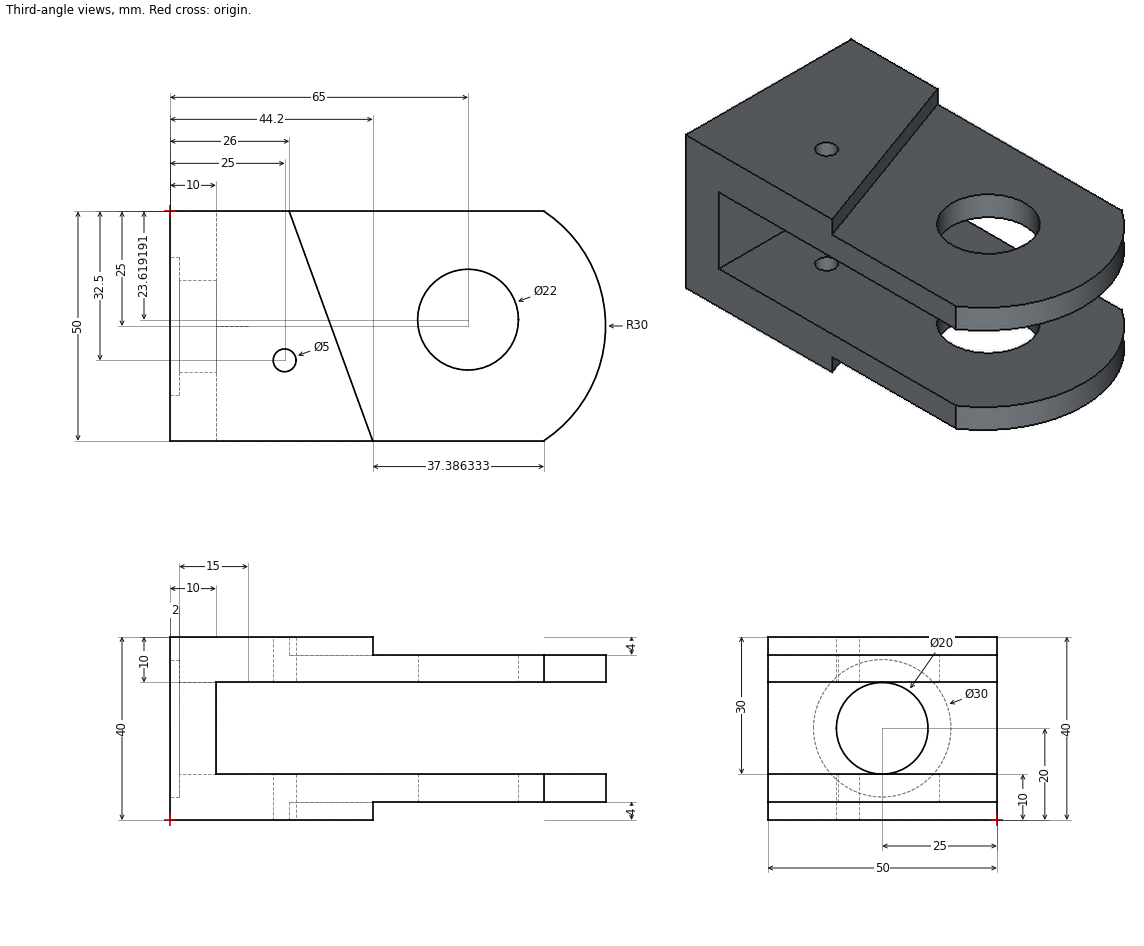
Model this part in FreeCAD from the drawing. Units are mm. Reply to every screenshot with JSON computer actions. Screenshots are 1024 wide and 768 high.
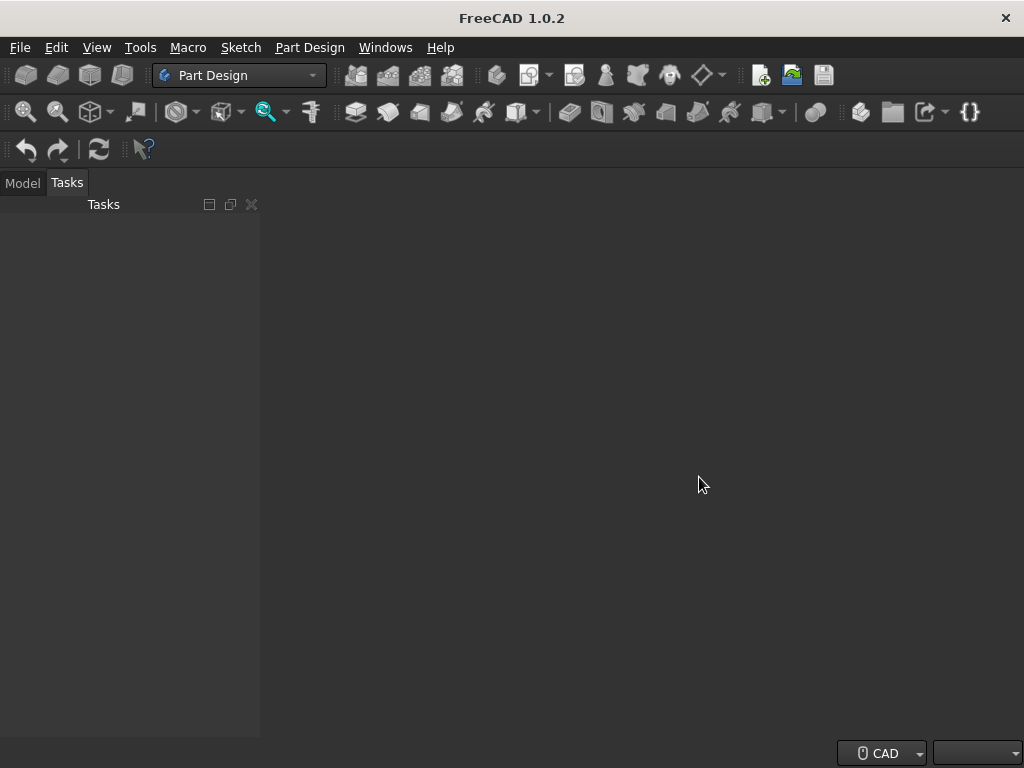
{"action": "left_click", "coordinate": [760, 76]}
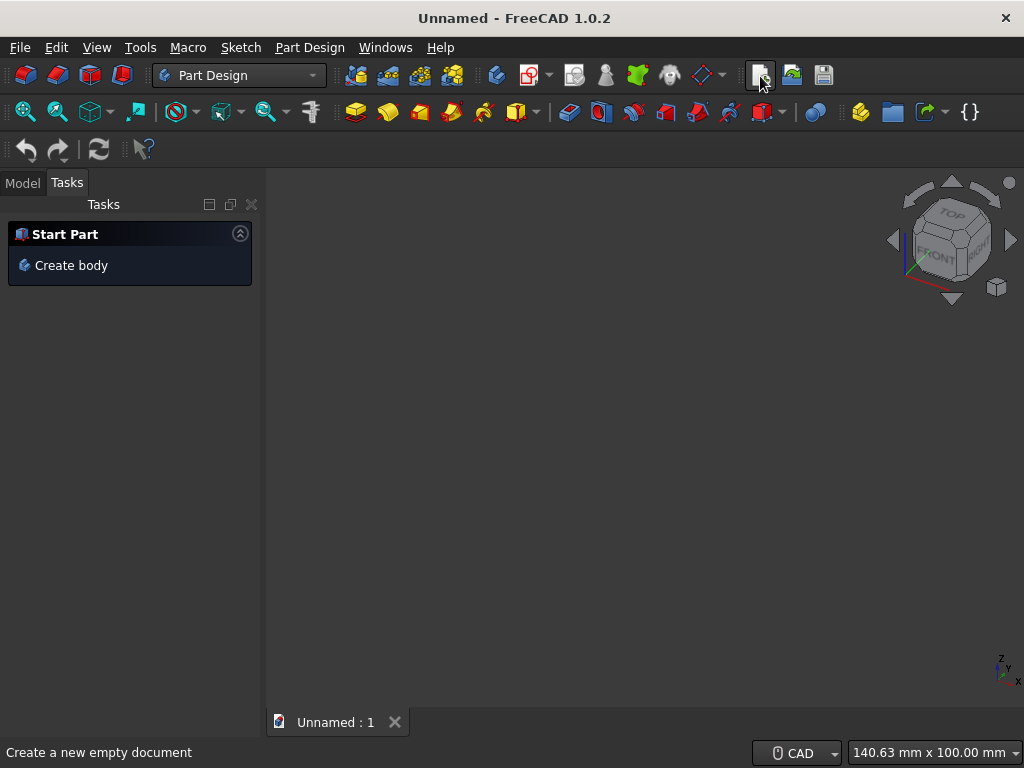
{"action": "left_click", "coordinate": [530, 76]}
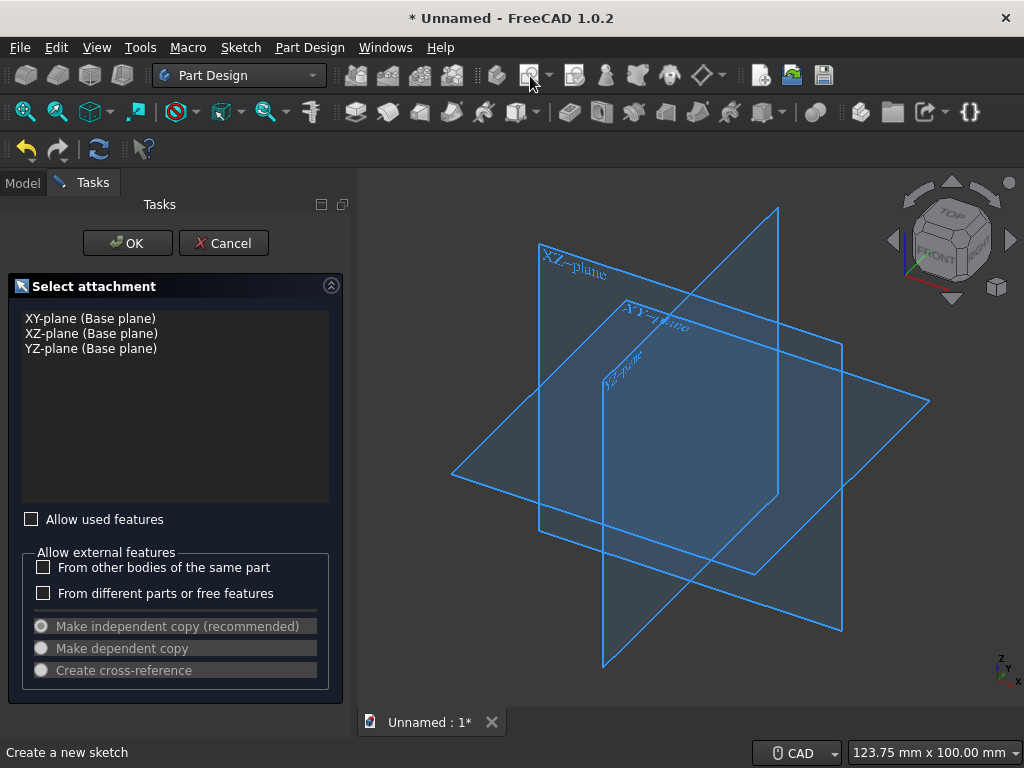
{"action": "left_click", "coordinate": [82, 318]}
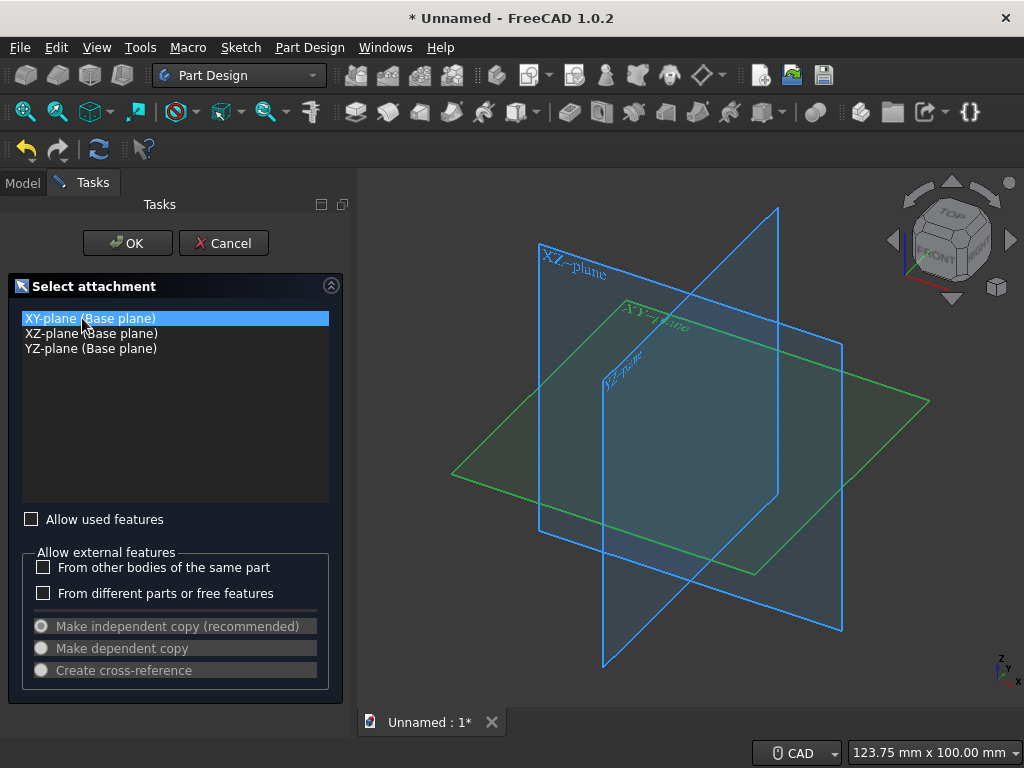
{"action": "left_click", "coordinate": [128, 243]}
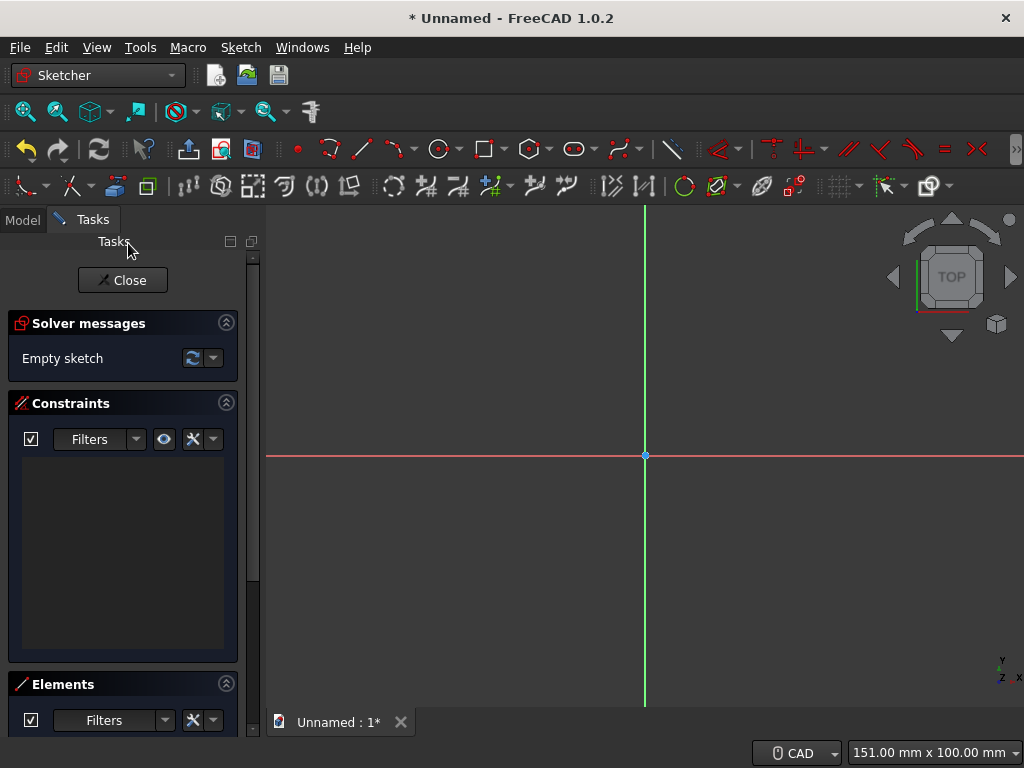
{"action": "scroll", "coordinate": [294, 303], "scroll_direction": "down", "scroll_amount": 3}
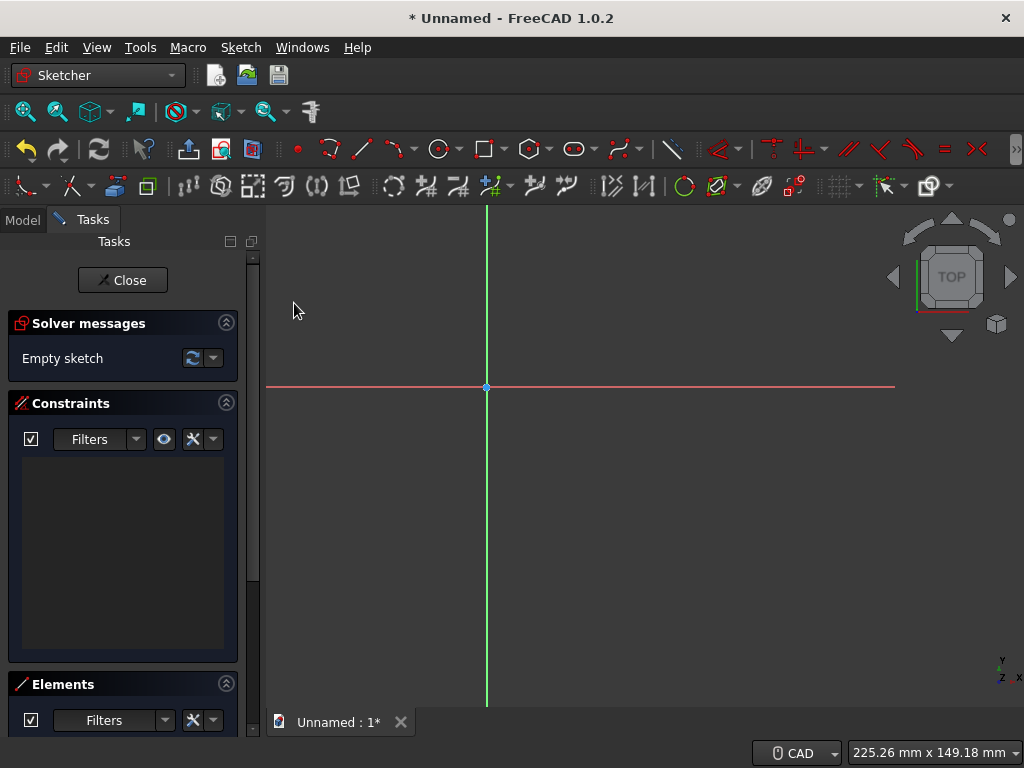
{"action": "scroll", "coordinate": [701, 456], "scroll_direction": "up", "scroll_amount": 2}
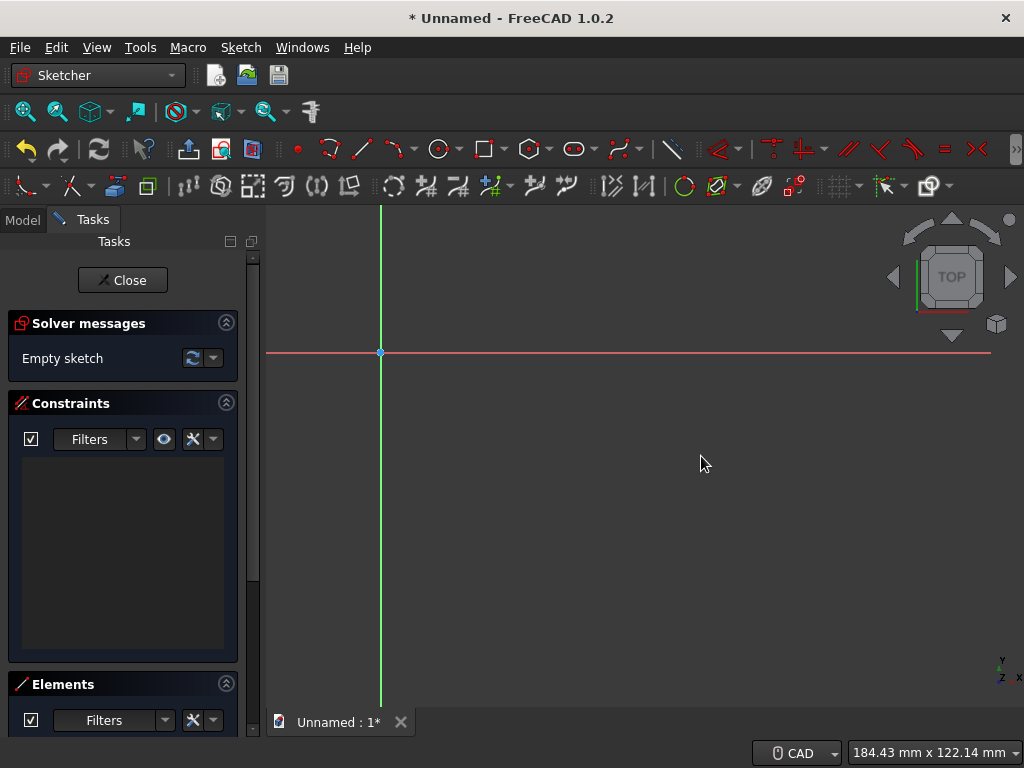
{"action": "key", "text": "g m"}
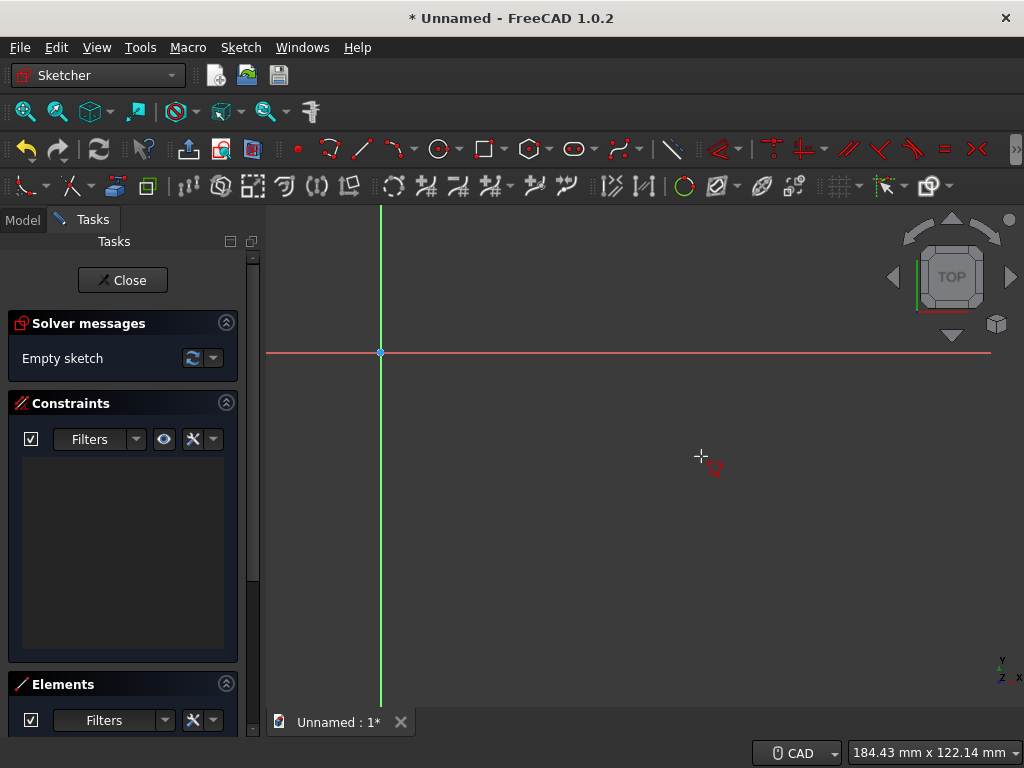
{"action": "left_click", "coordinate": [716, 353]}
{"action": "left_click", "coordinate": [381, 353]}
{"action": "left_click", "coordinate": [390, 558]}
{"action": "left_click", "coordinate": [716, 558]}
{"action": "right_click", "coordinate": [716, 558]}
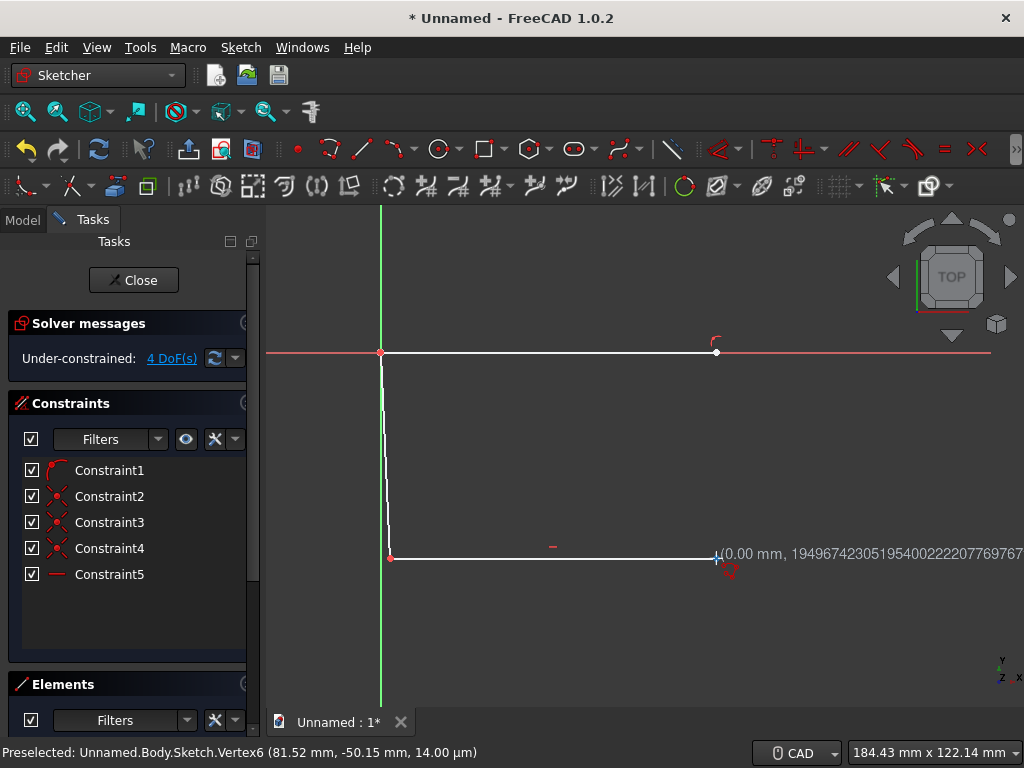
{"action": "left_click", "coordinate": [394, 150]}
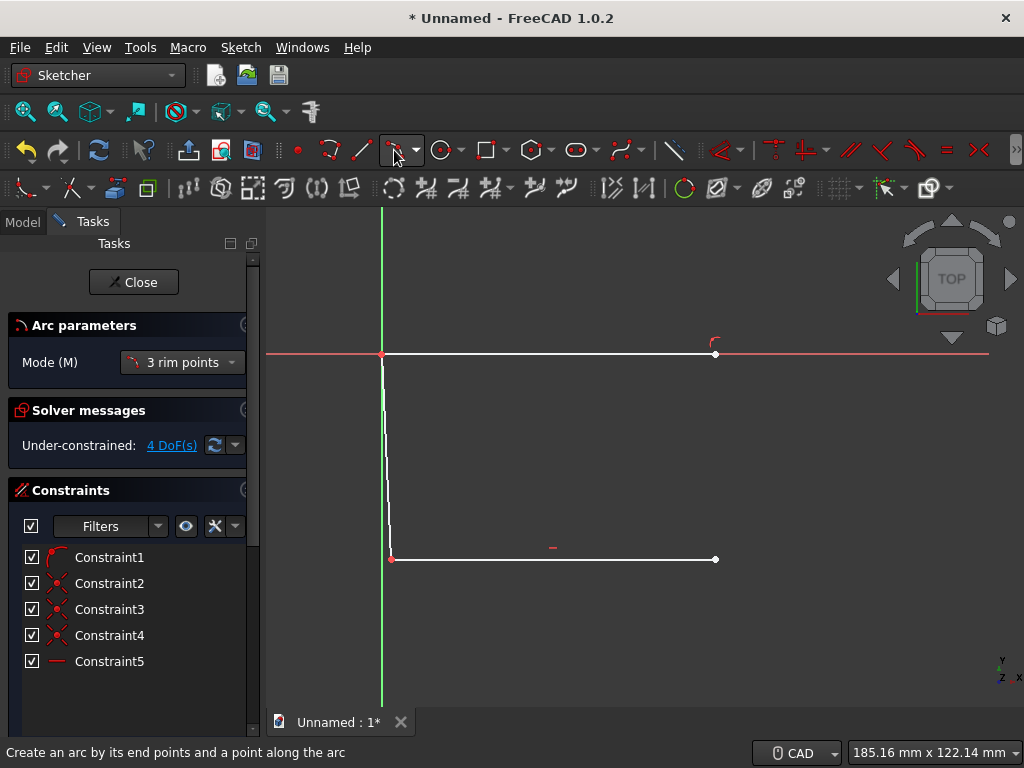
{"action": "left_click", "coordinate": [716, 560]}
{"action": "left_click", "coordinate": [716, 354]}
{"action": "left_click", "coordinate": [771, 457]}
{"action": "key", "text": "Escape"}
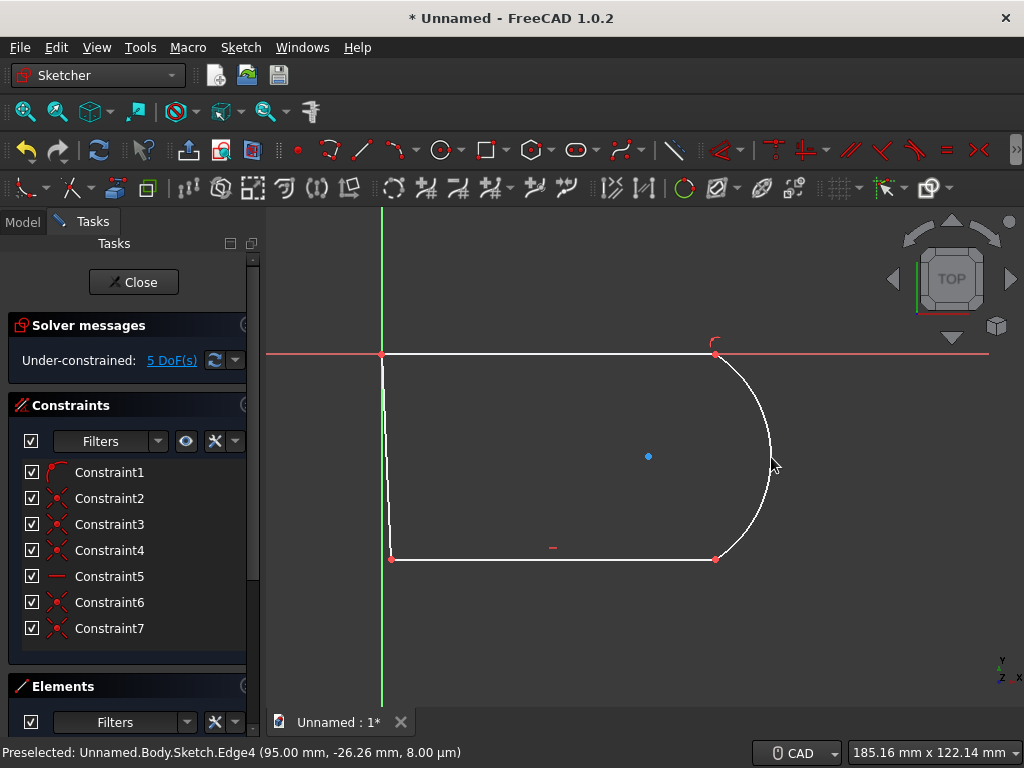
{"action": "left_click", "coordinate": [385, 416]}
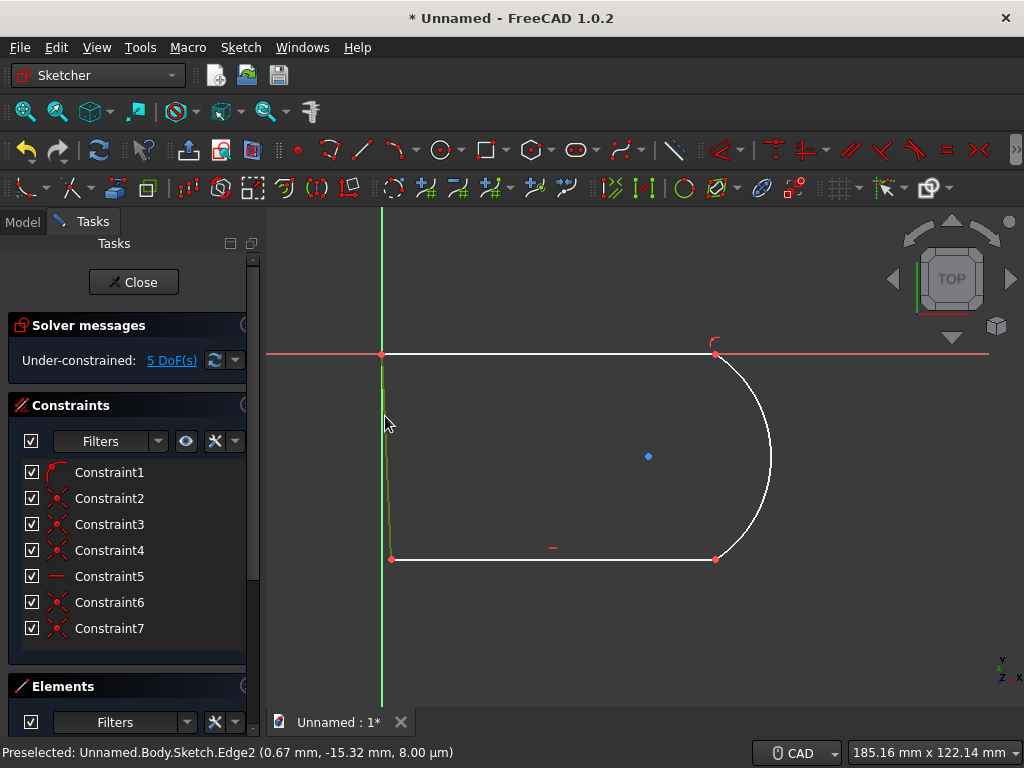
{"action": "key", "text": "v"}